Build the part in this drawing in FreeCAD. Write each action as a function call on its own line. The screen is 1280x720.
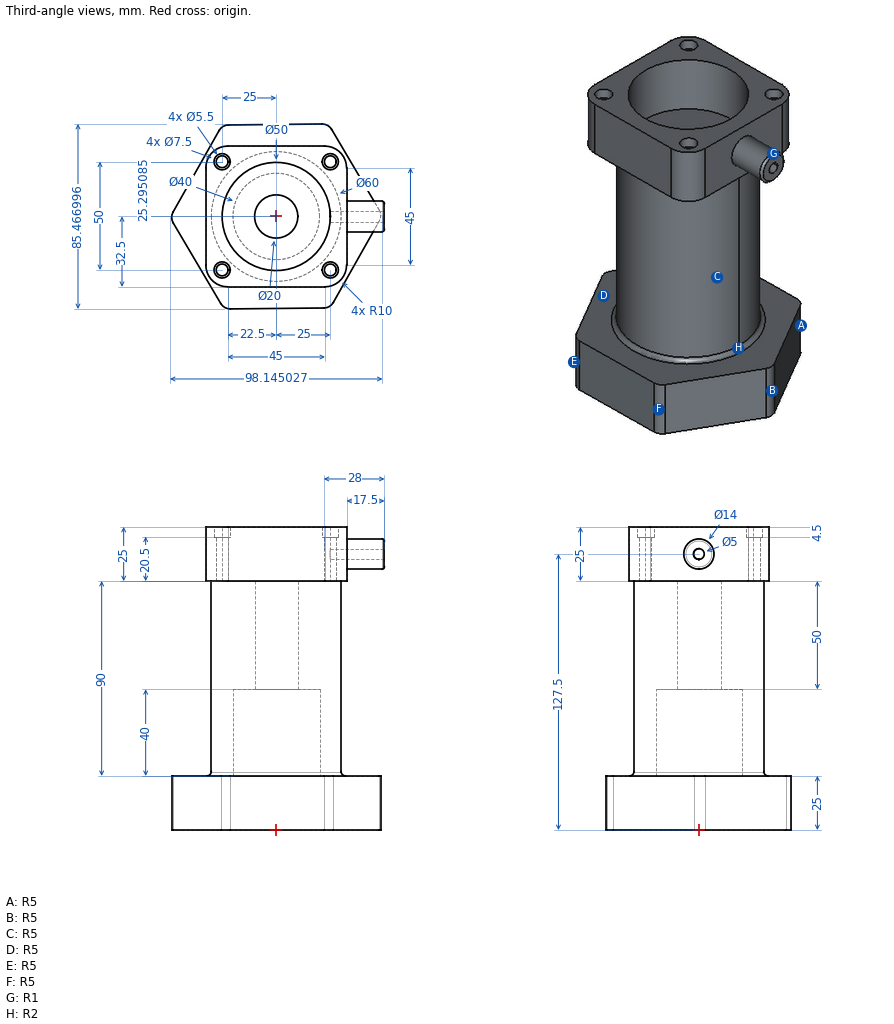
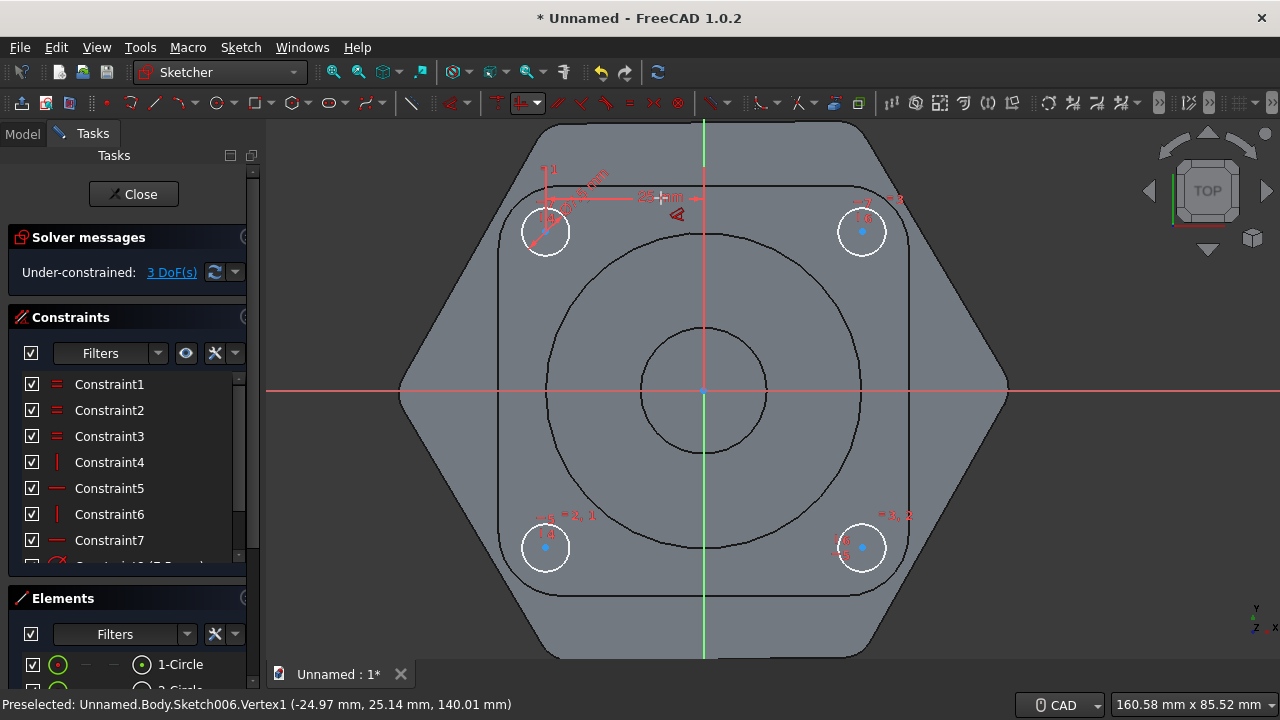
click(862, 548)
click(783, 582)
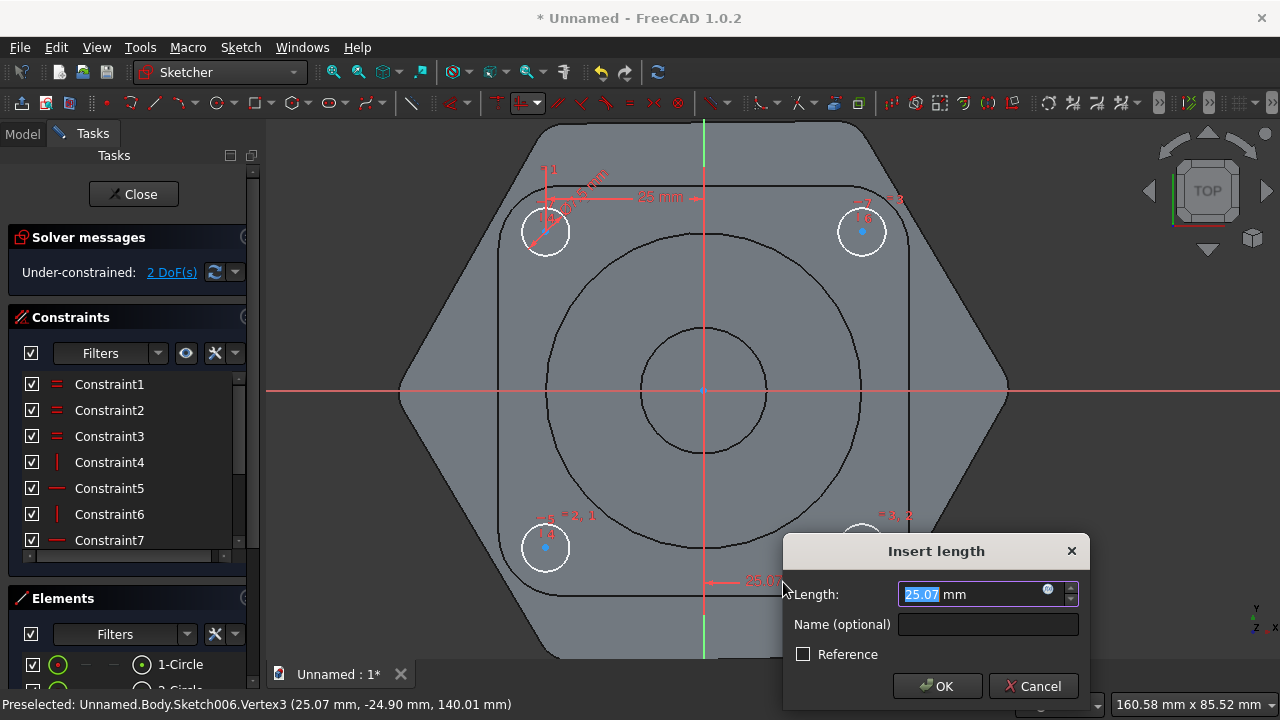
text(25)
key(Return)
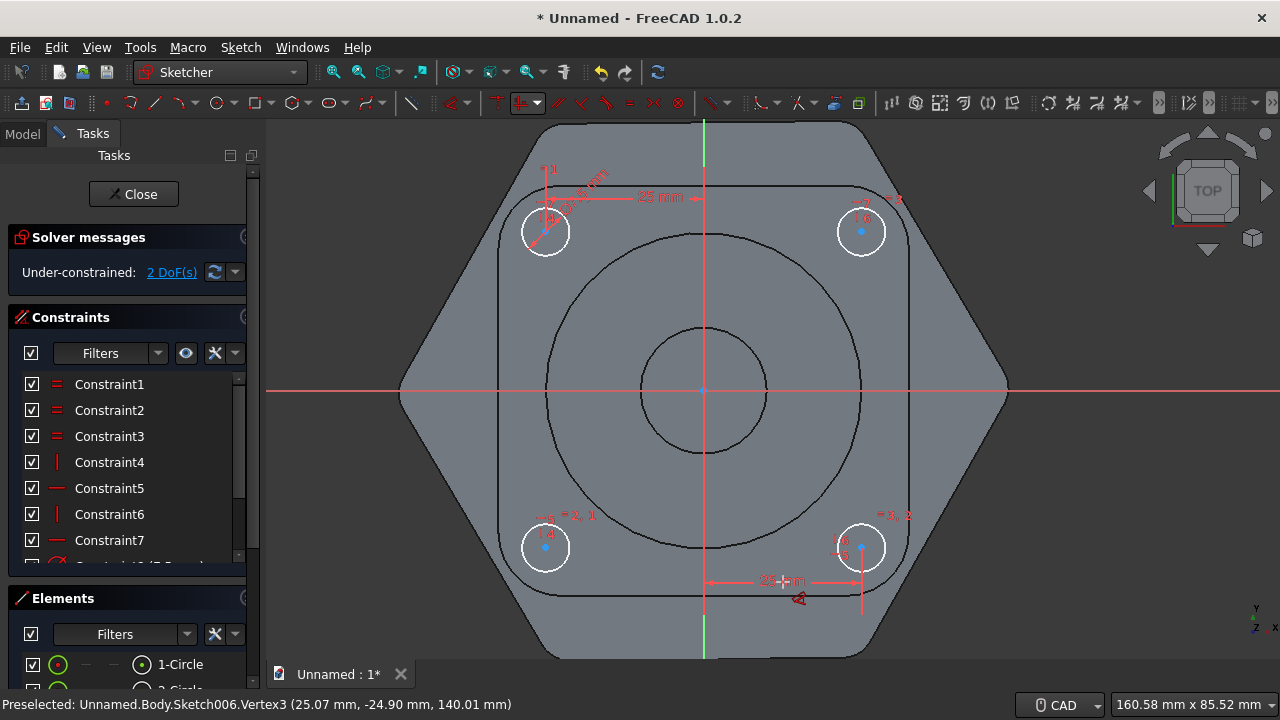
click(546, 232)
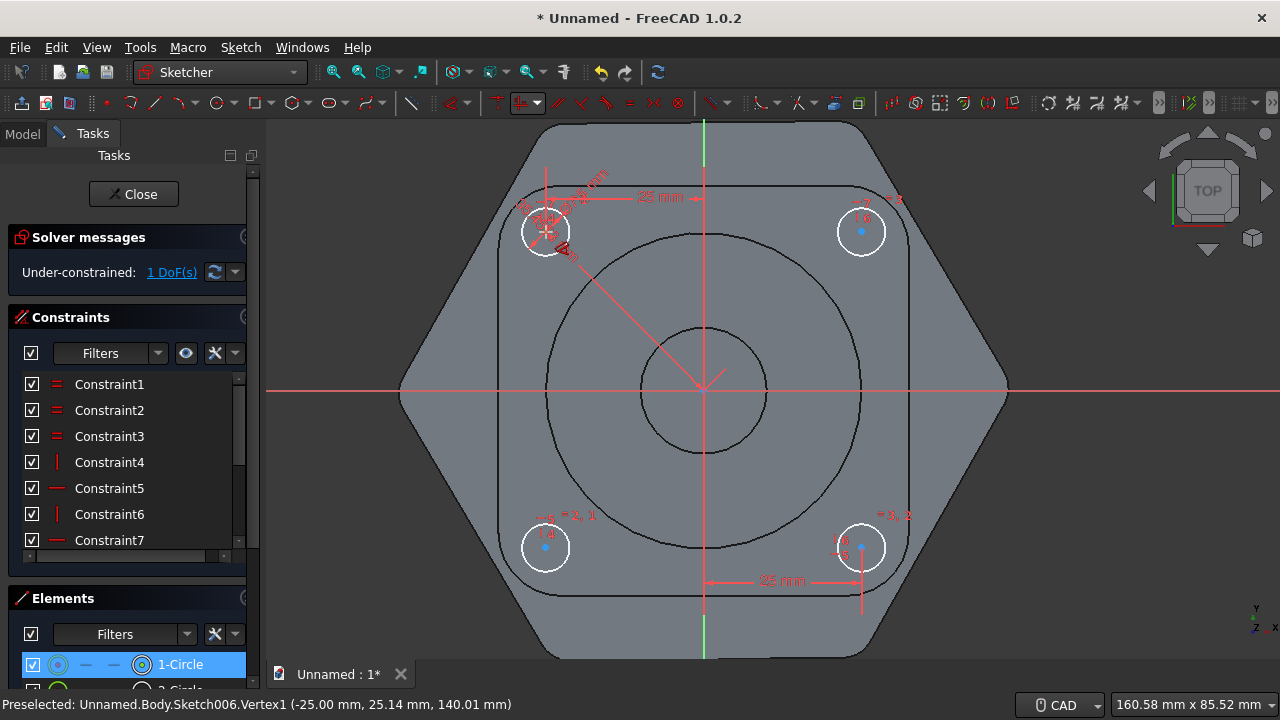
click(546, 548)
click(512, 317)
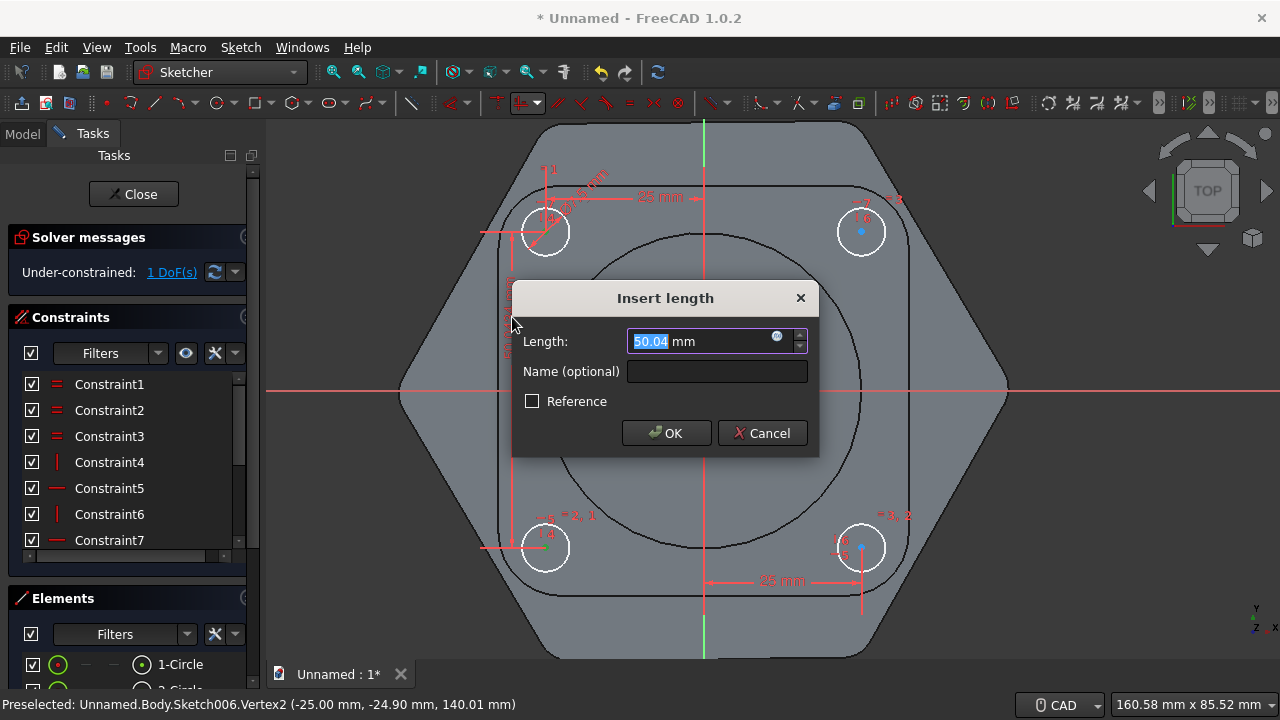
text(50)
key(Return)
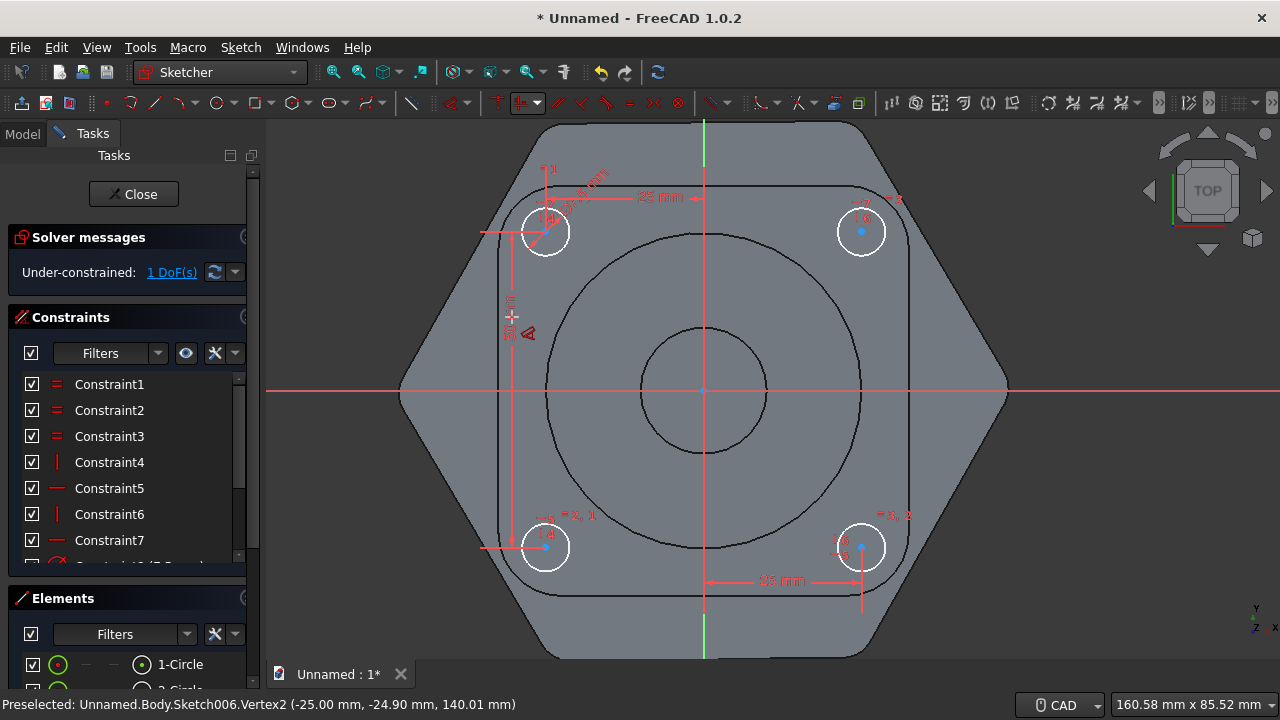
click(546, 232)
click(512, 275)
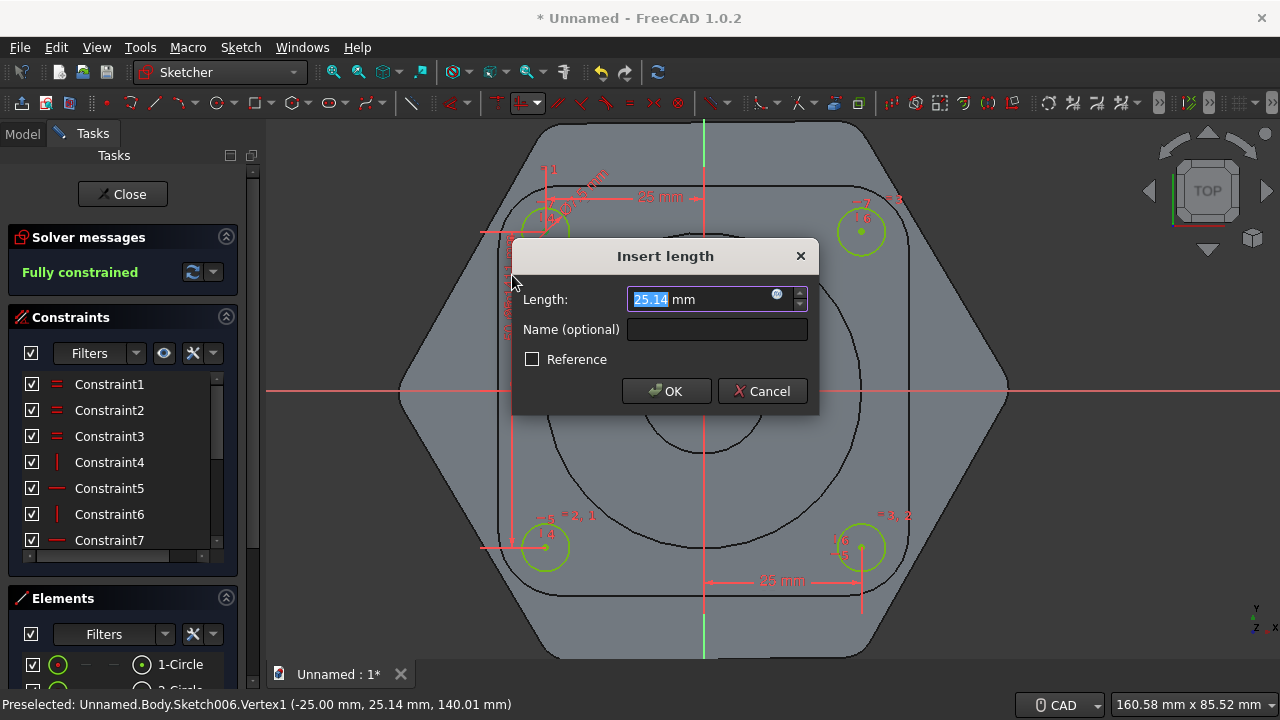
text(25.295085)
key(Return)
key(Escape)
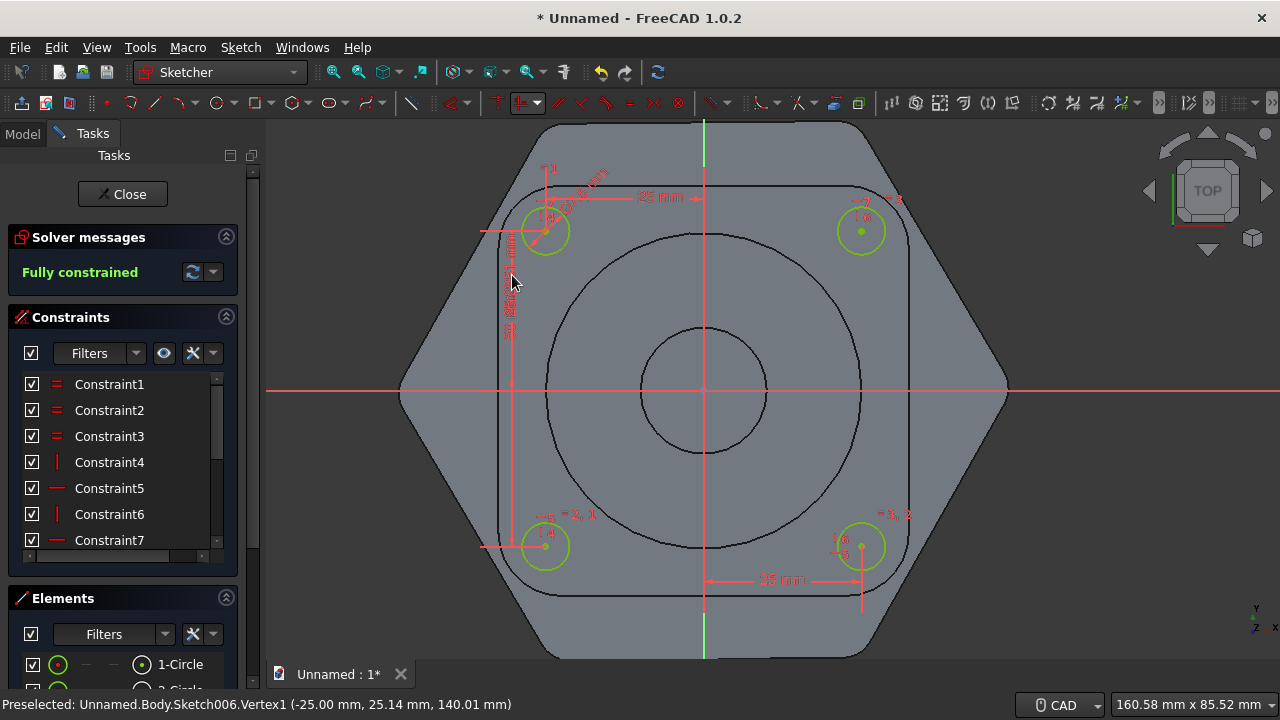
click(123, 194)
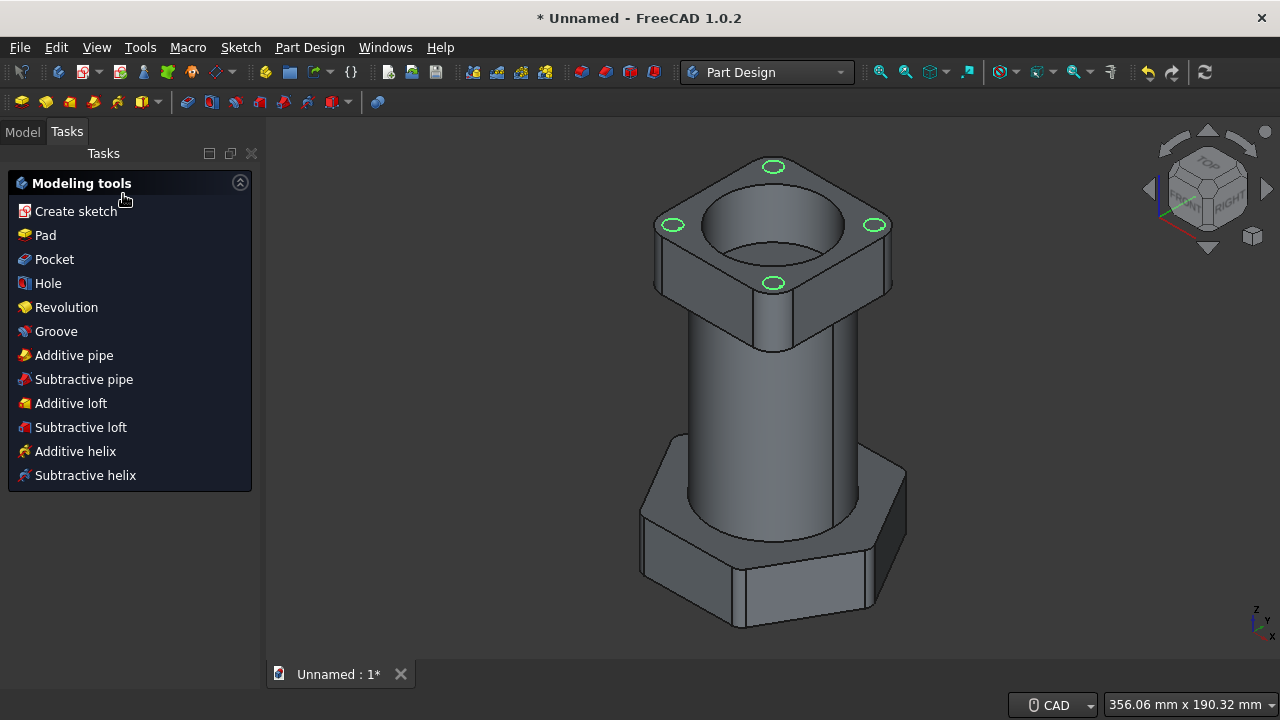
click(188, 102)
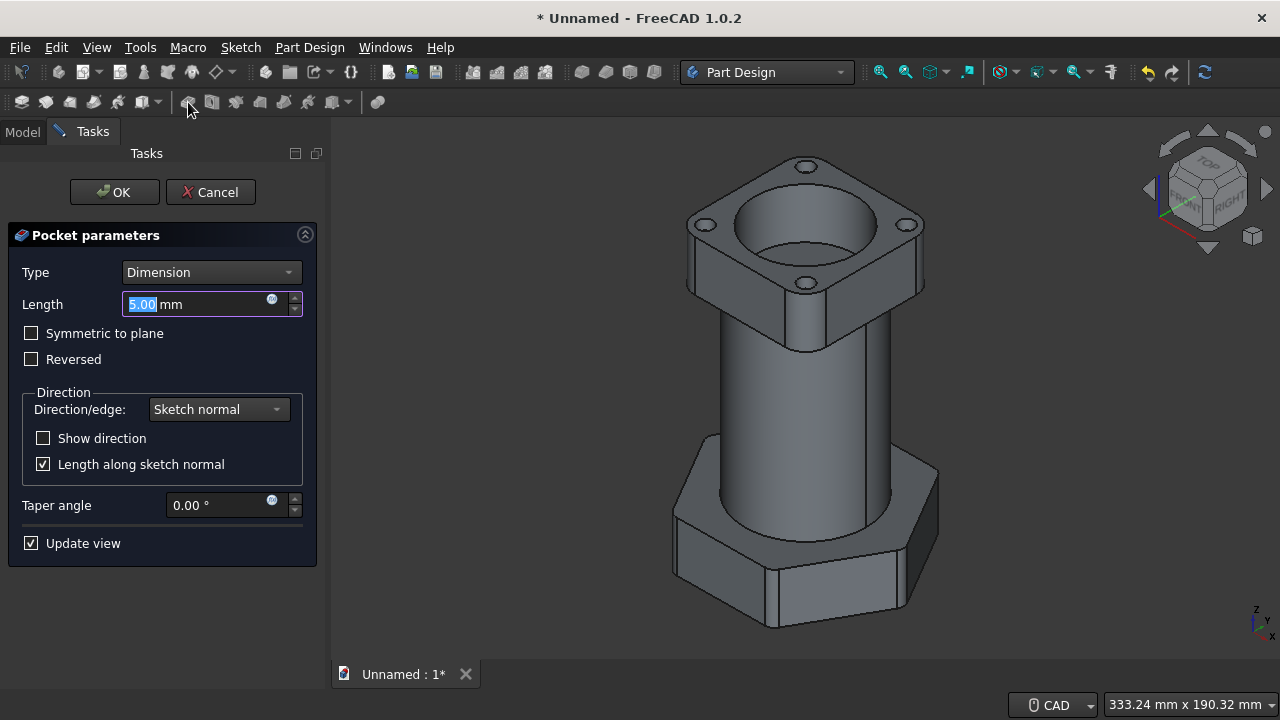
text(4.5)
key(Tab)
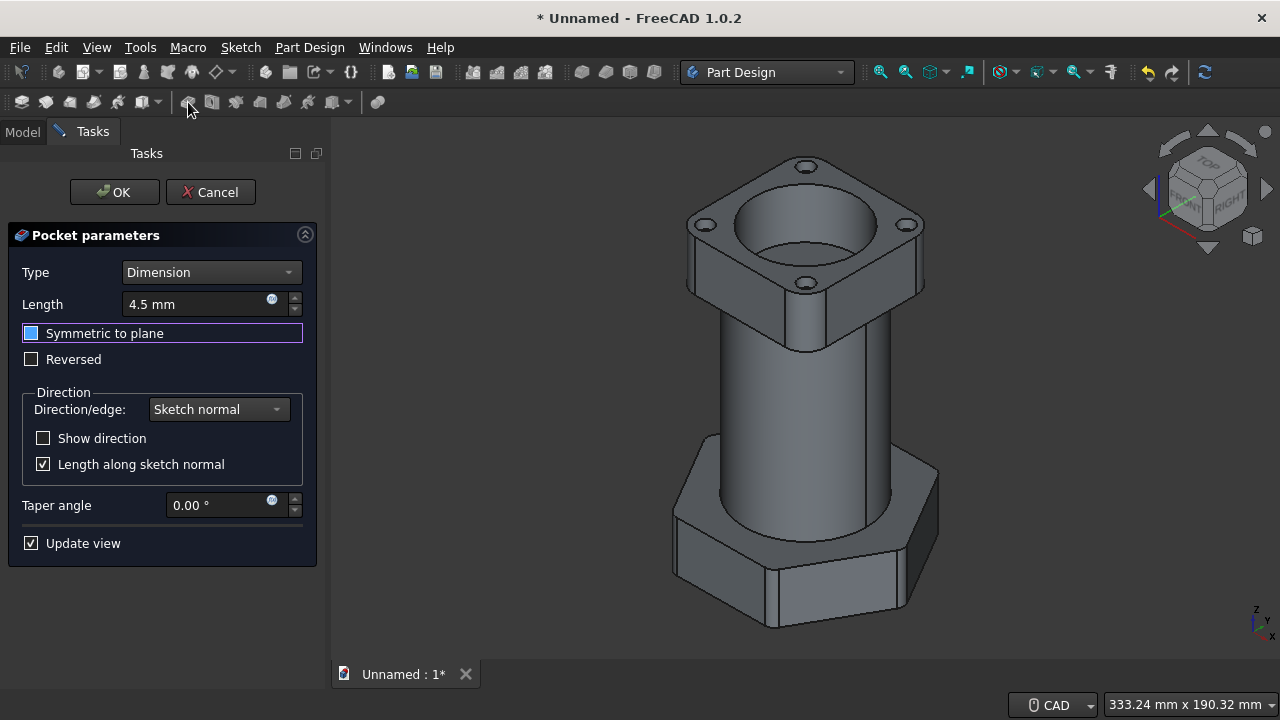
click(115, 192)